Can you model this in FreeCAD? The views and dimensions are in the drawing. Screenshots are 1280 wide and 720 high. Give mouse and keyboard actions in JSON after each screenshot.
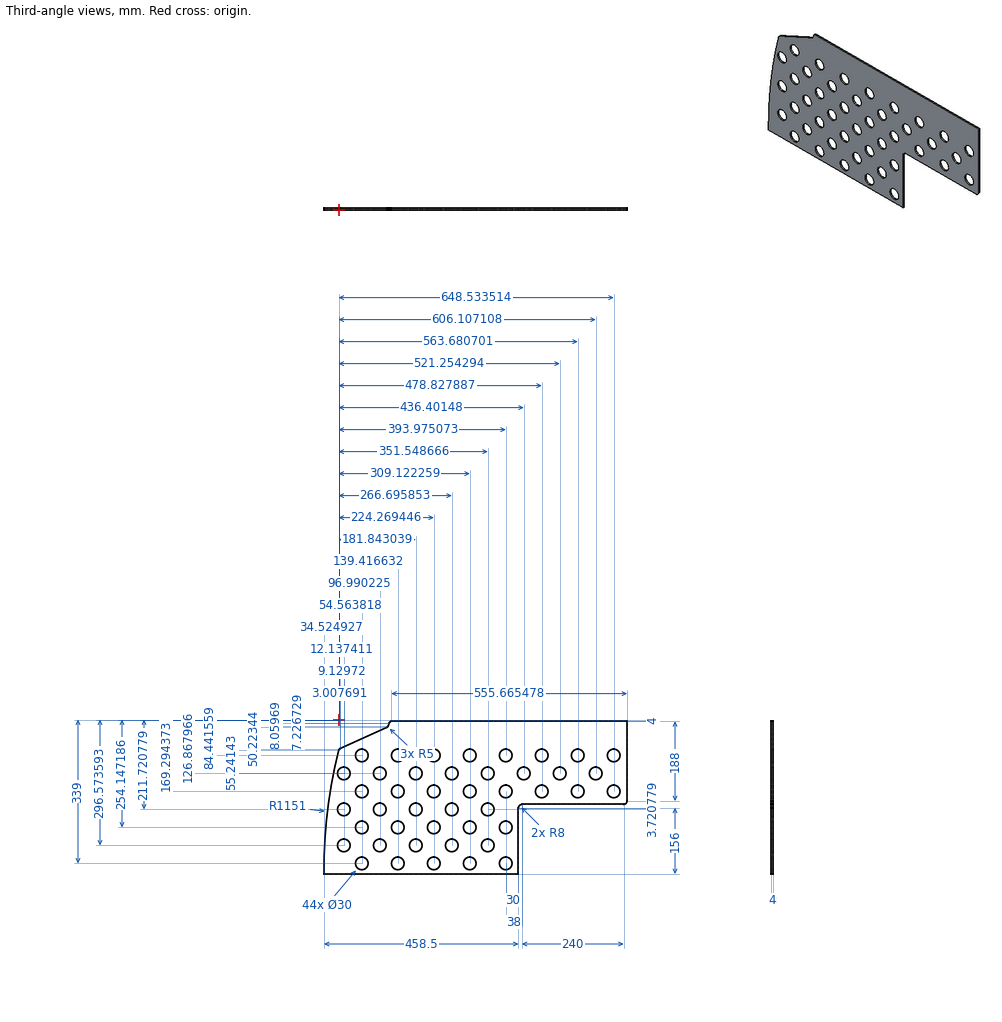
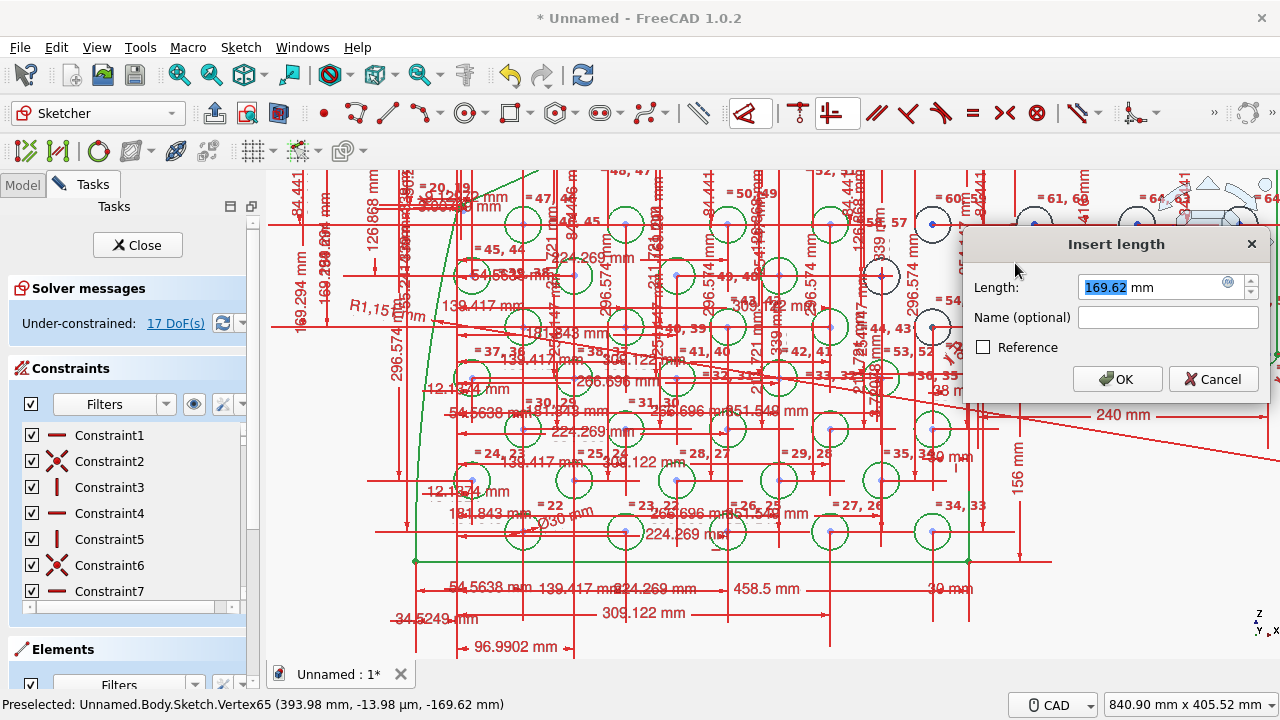
{"action": "type", "text": "169.294373"}
{"action": "key", "text": "Return"}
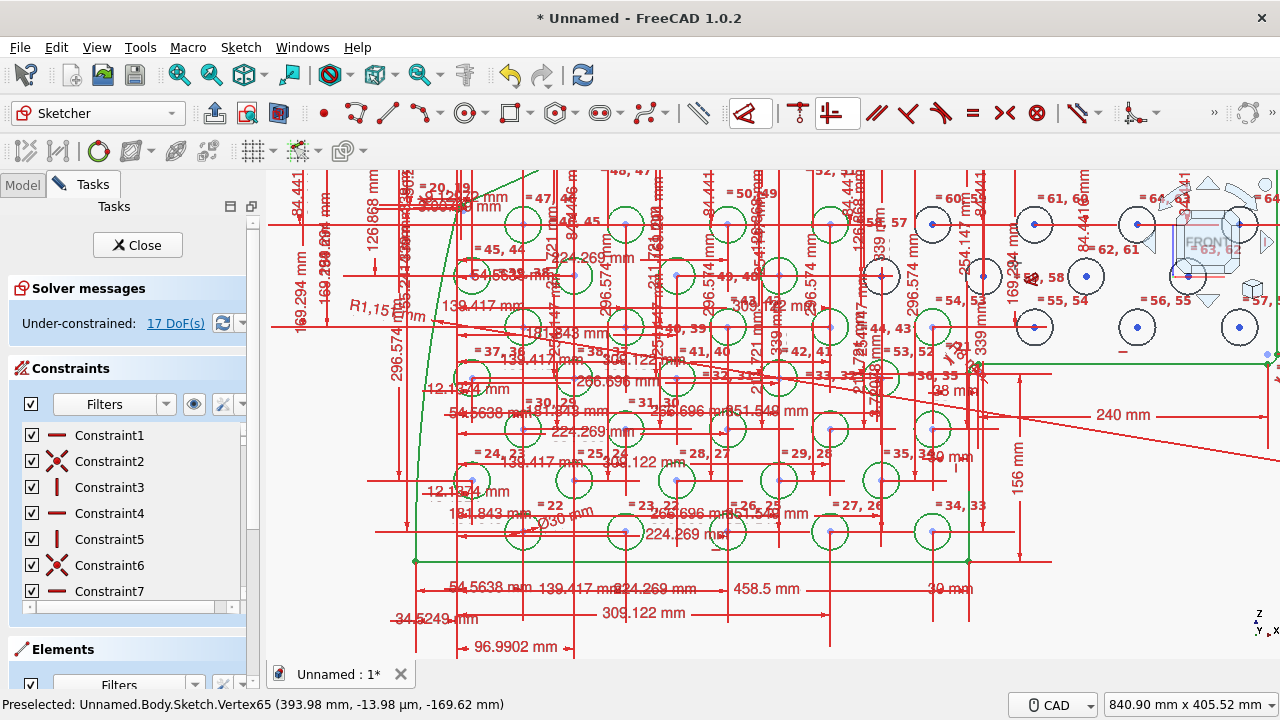
{"action": "left_click", "coordinate": [1035, 327]}
{"action": "left_click", "coordinate": [746, 385]}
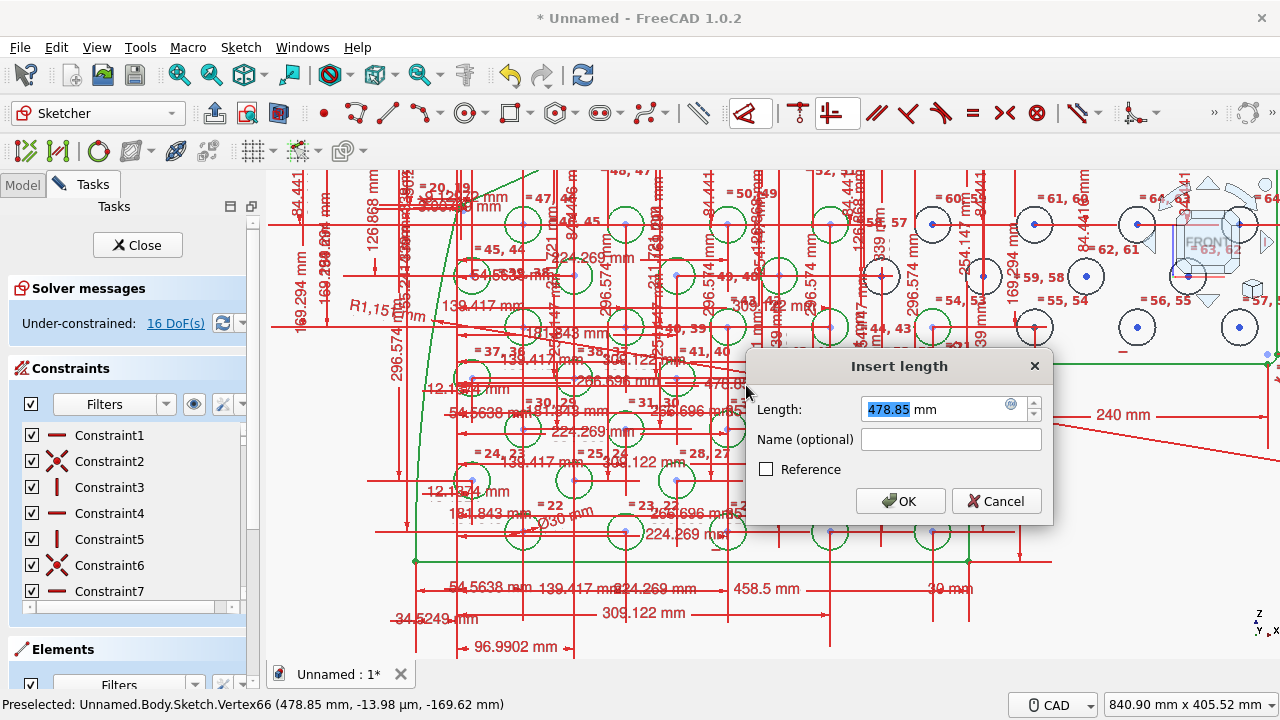
{"action": "type", "text": "478.827887"}
{"action": "key", "text": "Return"}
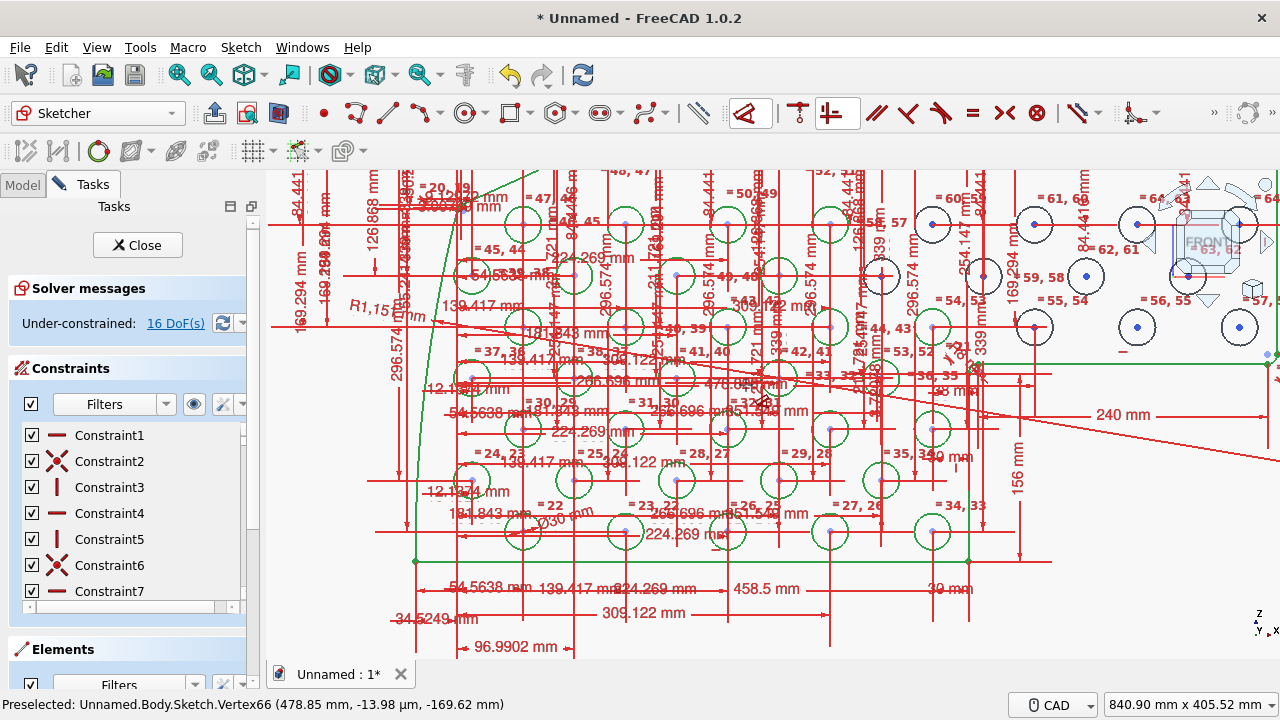
{"action": "left_click", "coordinate": [1035, 327]}
{"action": "left_click", "coordinate": [1069, 233]}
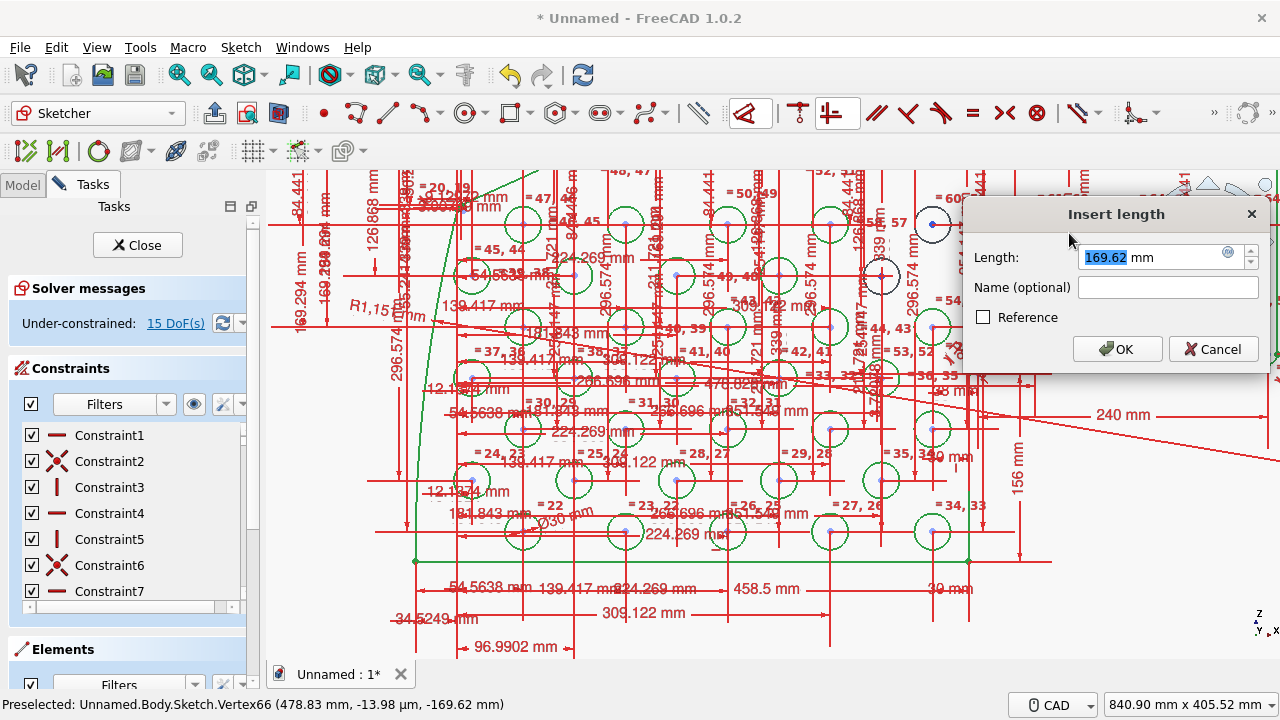
{"action": "type", "text": "169.294373"}
{"action": "key", "text": "Return"}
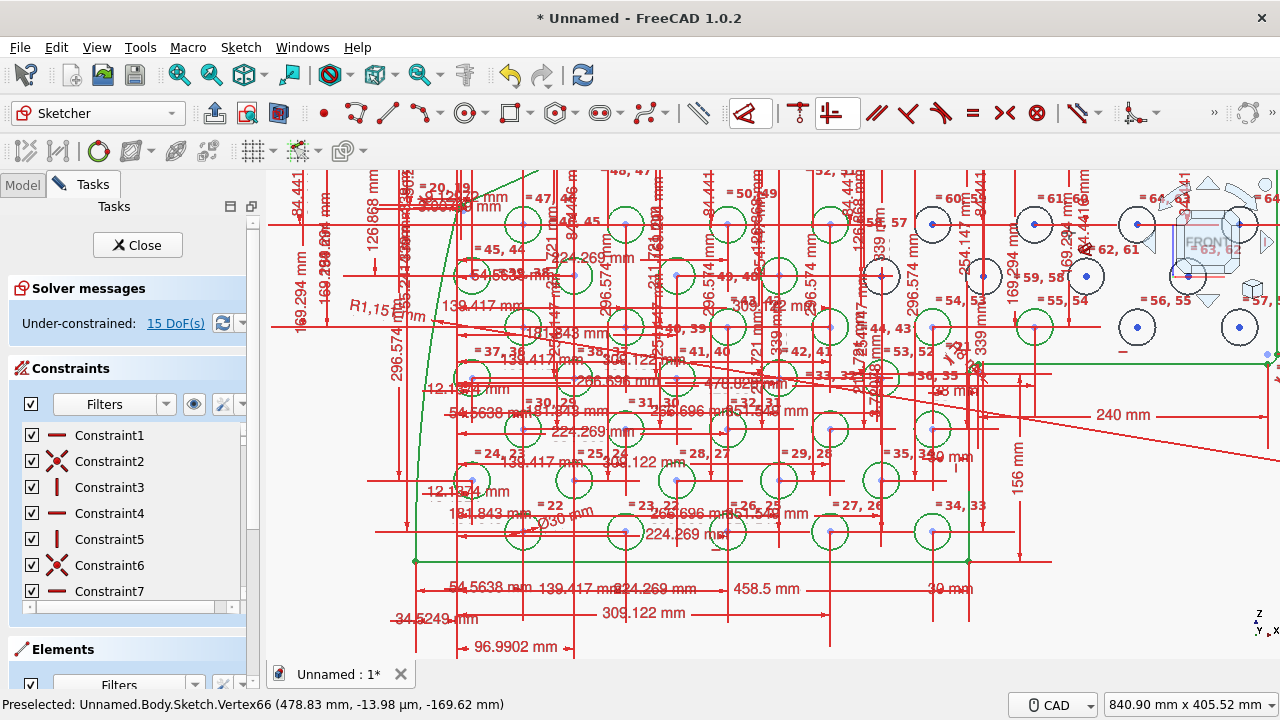
{"action": "scroll", "coordinate": [416, 561], "scroll_direction": "down", "scroll_amount": 2}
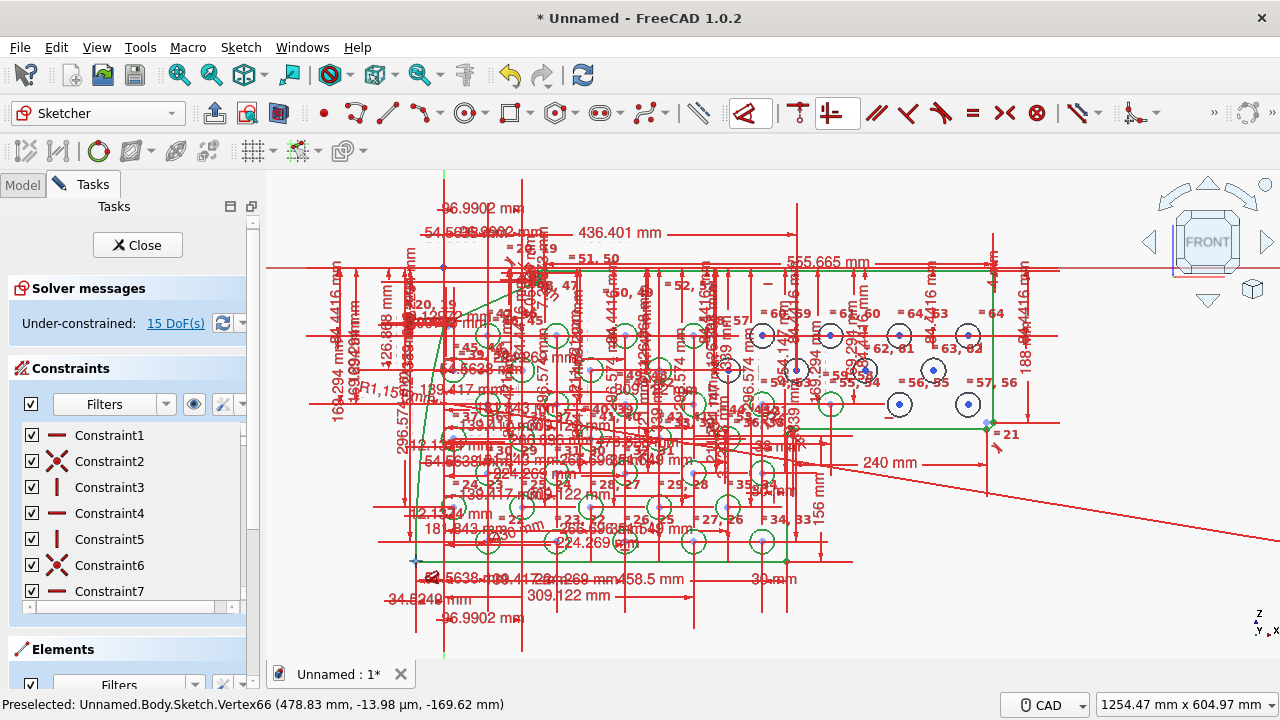
{"action": "left_click", "coordinate": [900, 405]}
{"action": "left_click", "coordinate": [777, 234]}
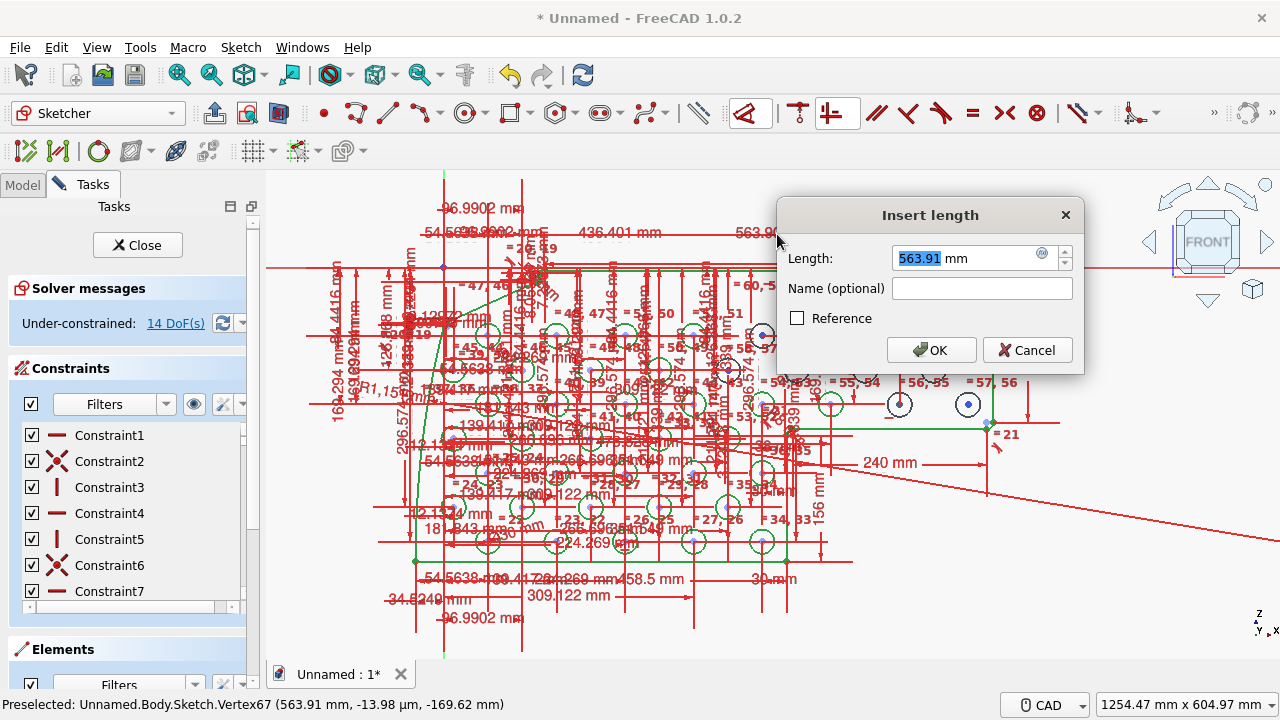
{"action": "type", "text": "563.680701"}
{"action": "key", "text": "Return"}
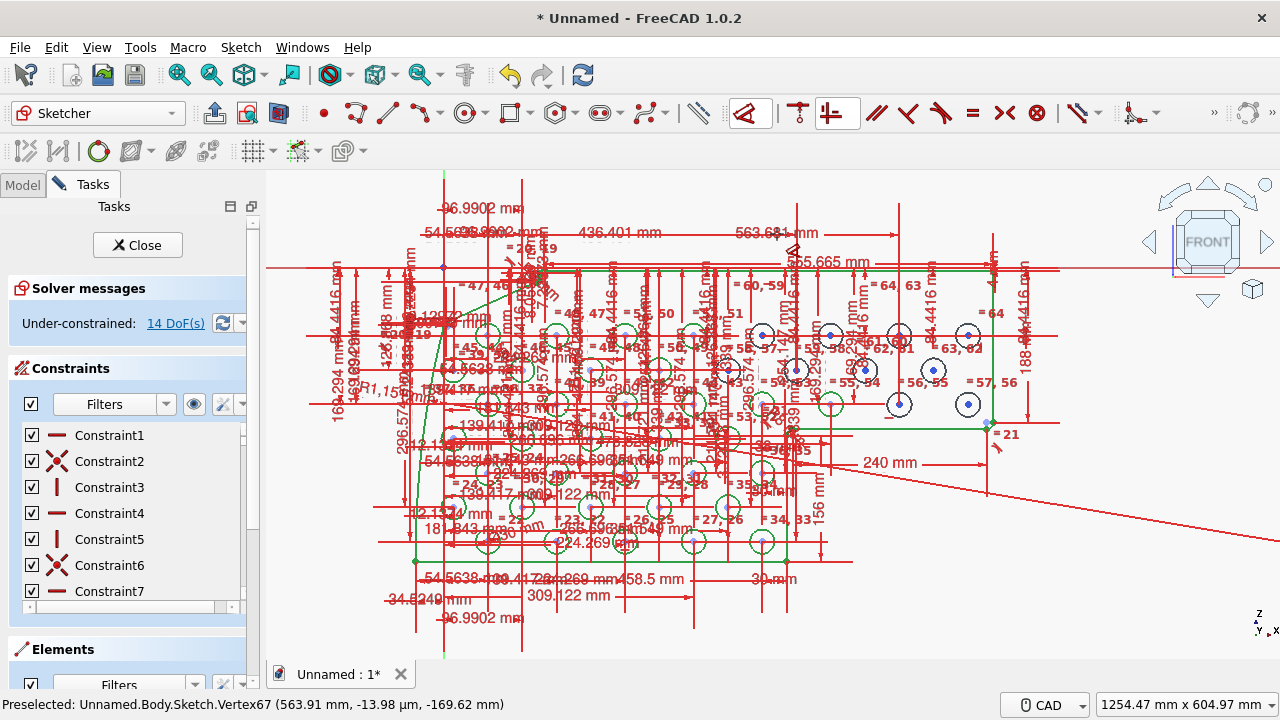
{"action": "left_click", "coordinate": [899, 405]}
{"action": "left_click", "coordinate": [1029, 368]}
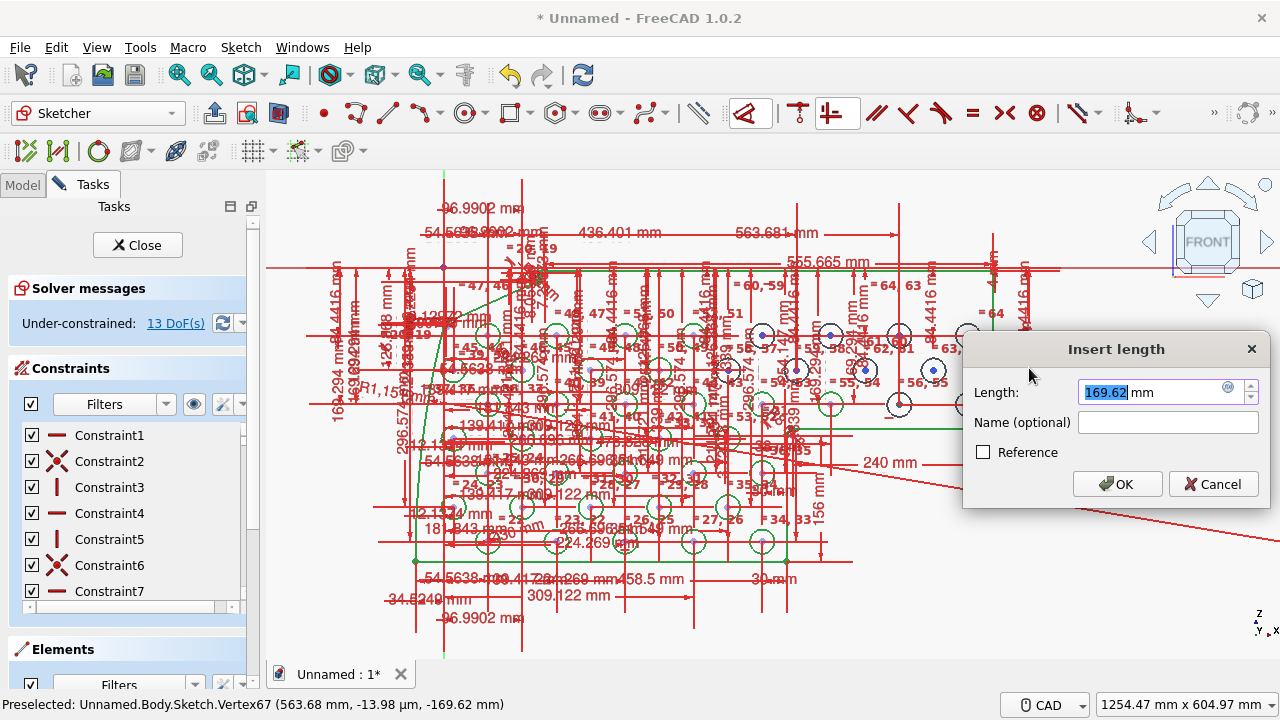
{"action": "type", "text": "169.294373"}
{"action": "key", "text": "Return"}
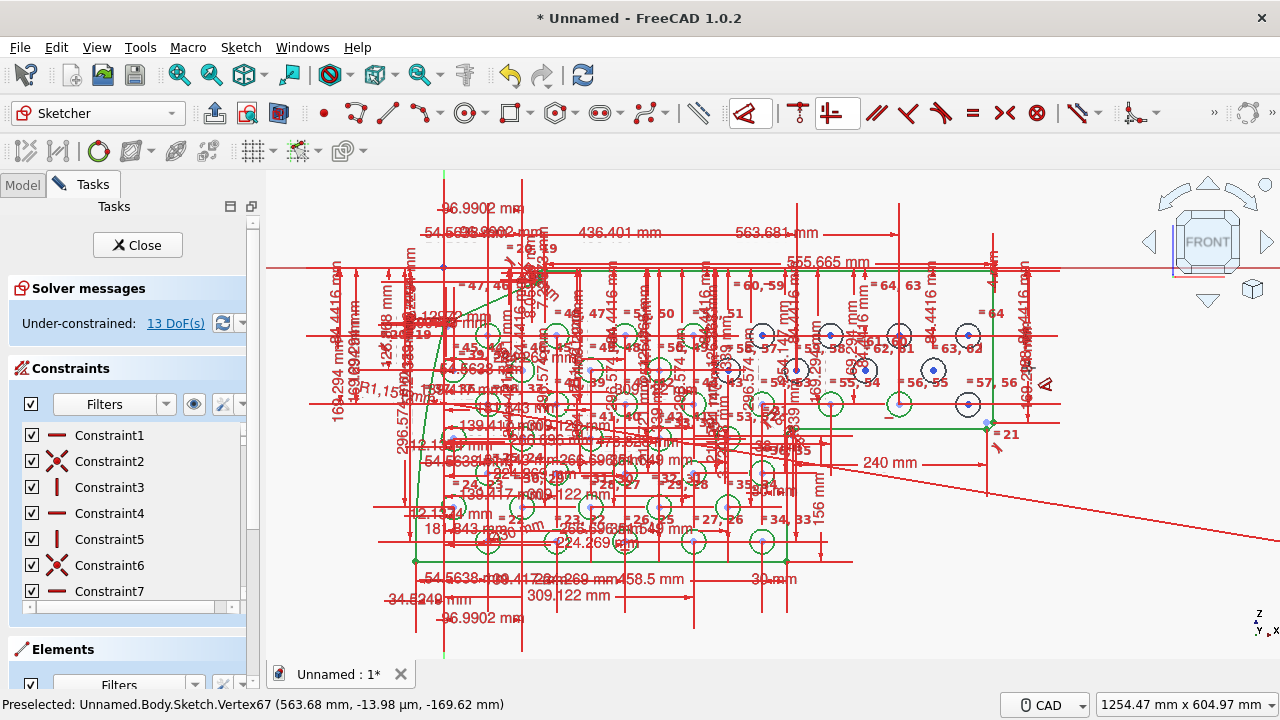
{"action": "left_click", "coordinate": [968, 405]}
{"action": "left_click", "coordinate": [706, 234]}